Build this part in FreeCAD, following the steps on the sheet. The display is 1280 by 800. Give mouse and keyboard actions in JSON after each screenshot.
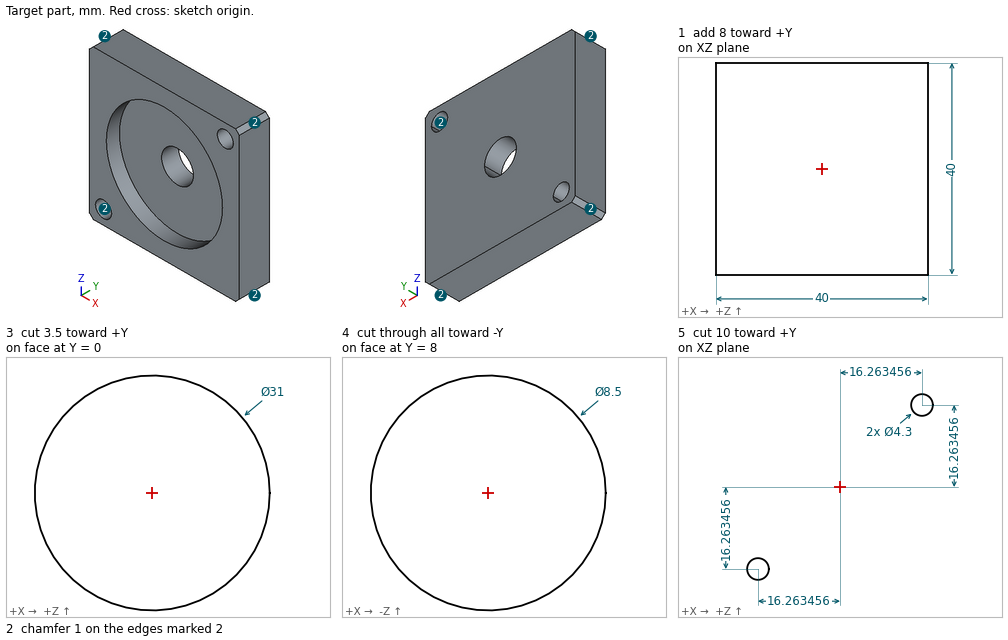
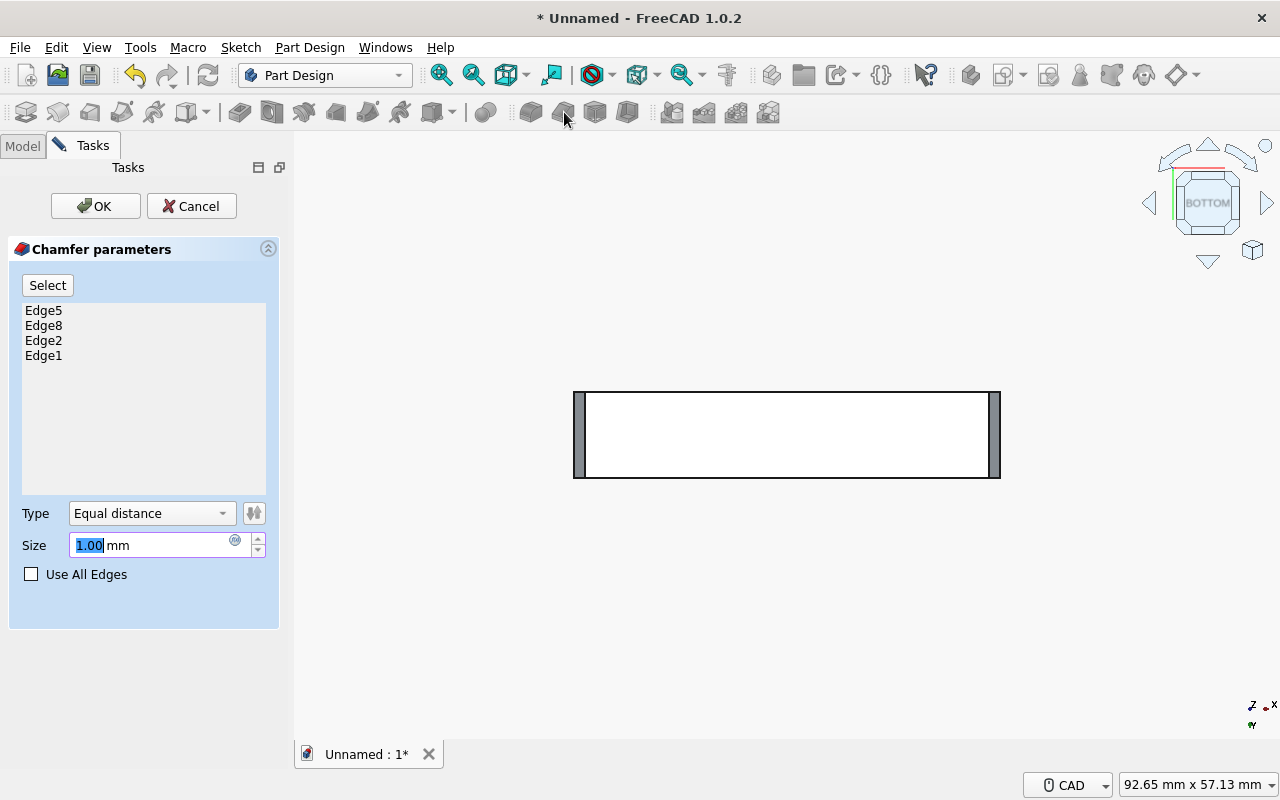
{"action": "type", "text": "1"}
{"action": "key", "text": "Tab"}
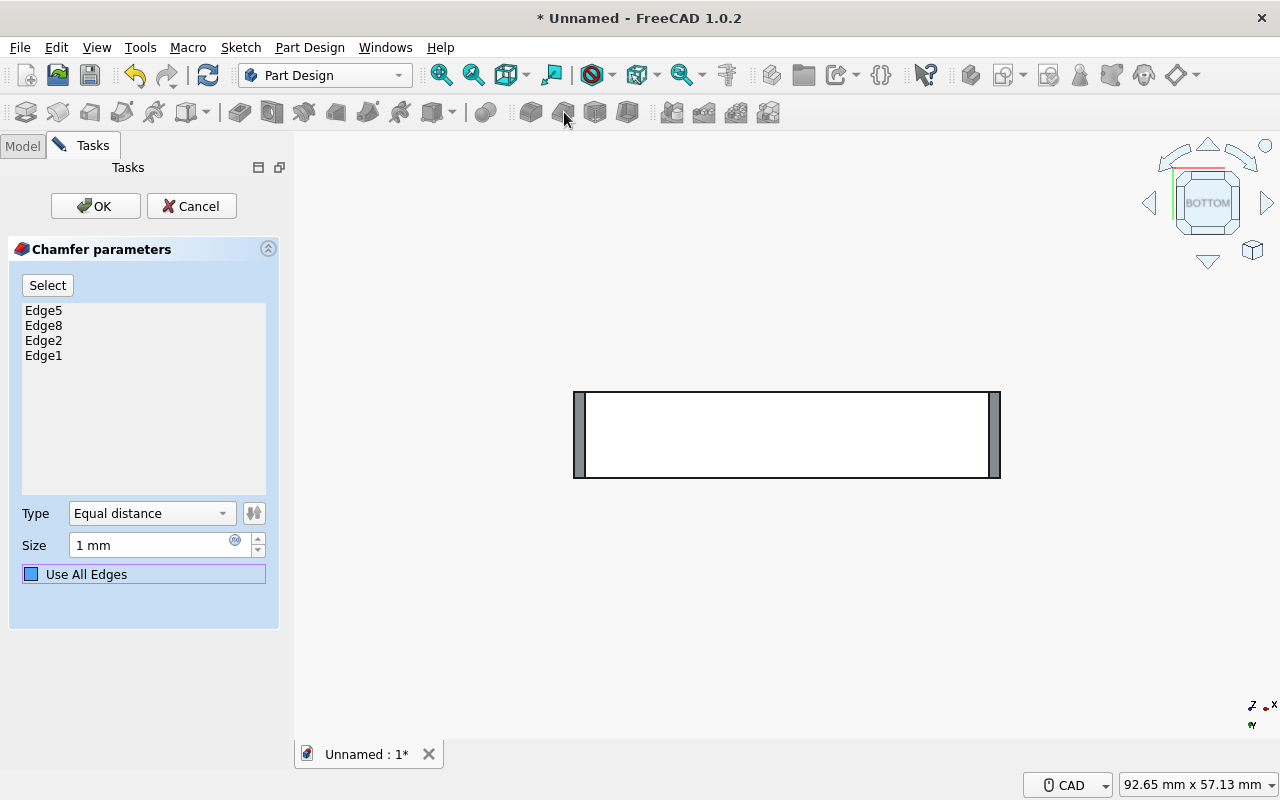
{"action": "left_click", "coordinate": [96, 206]}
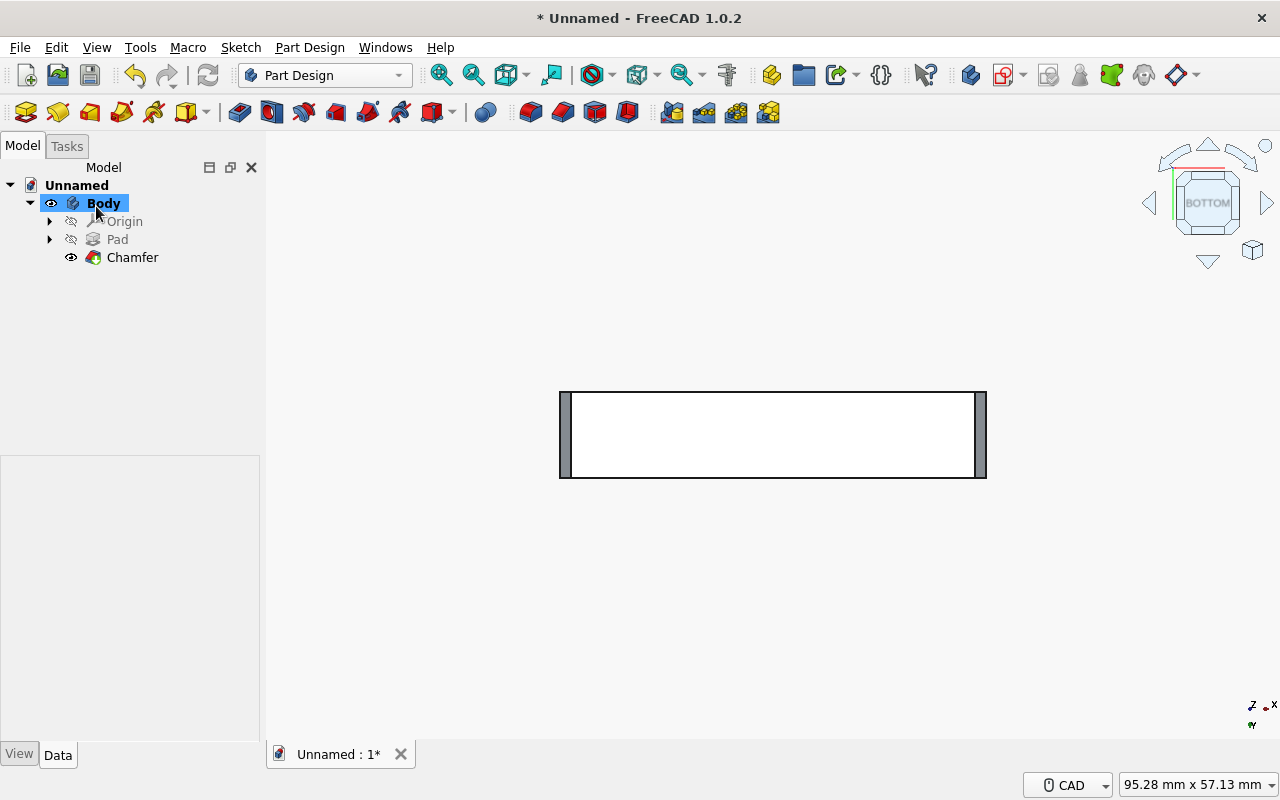
{"action": "left_click", "coordinate": [442, 76]}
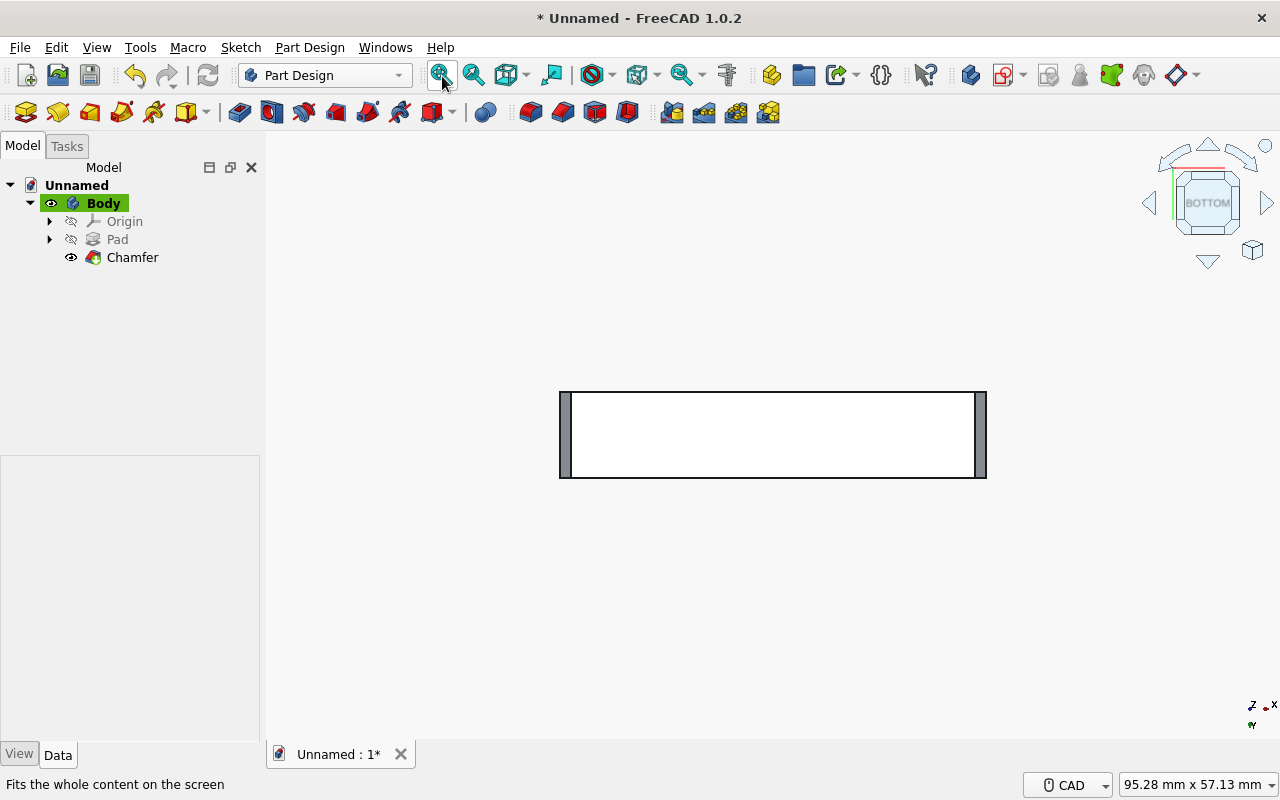
{"action": "key", "text": "0"}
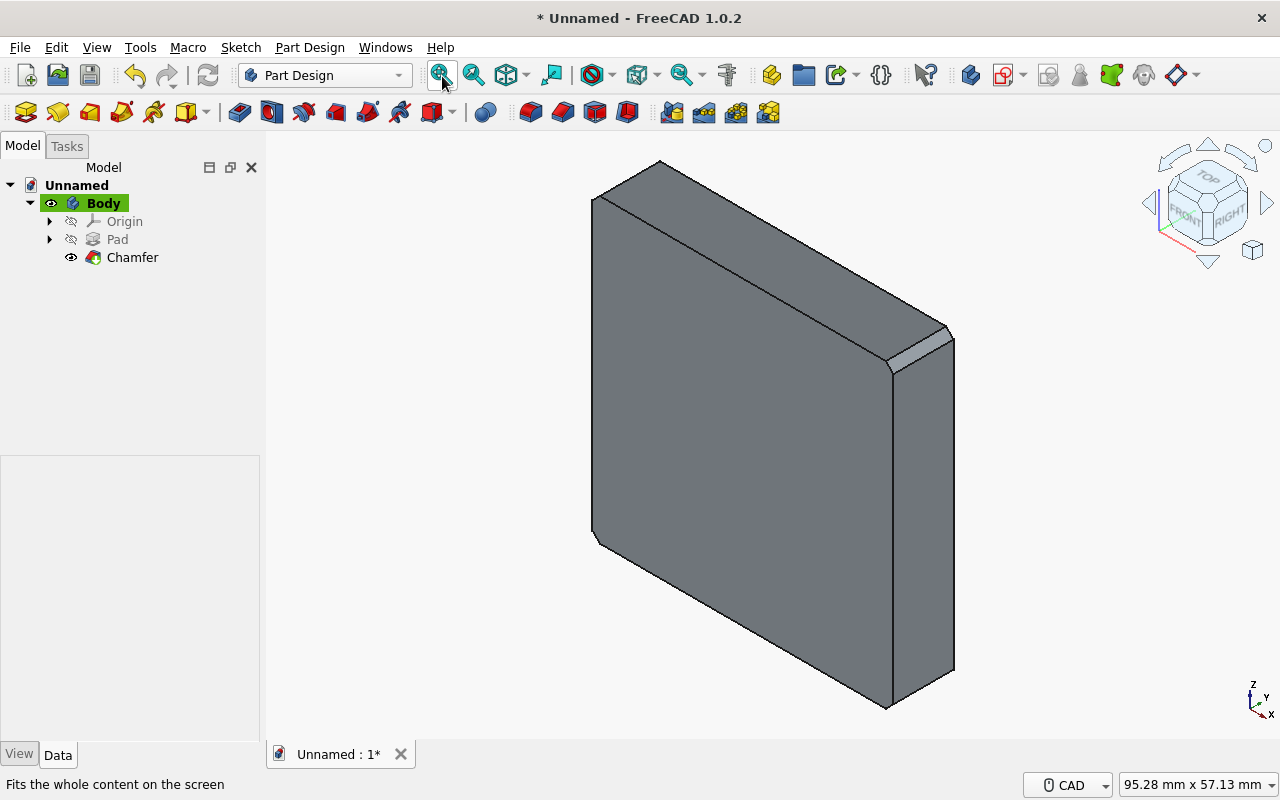
{"action": "left_click", "coordinate": [743, 451]}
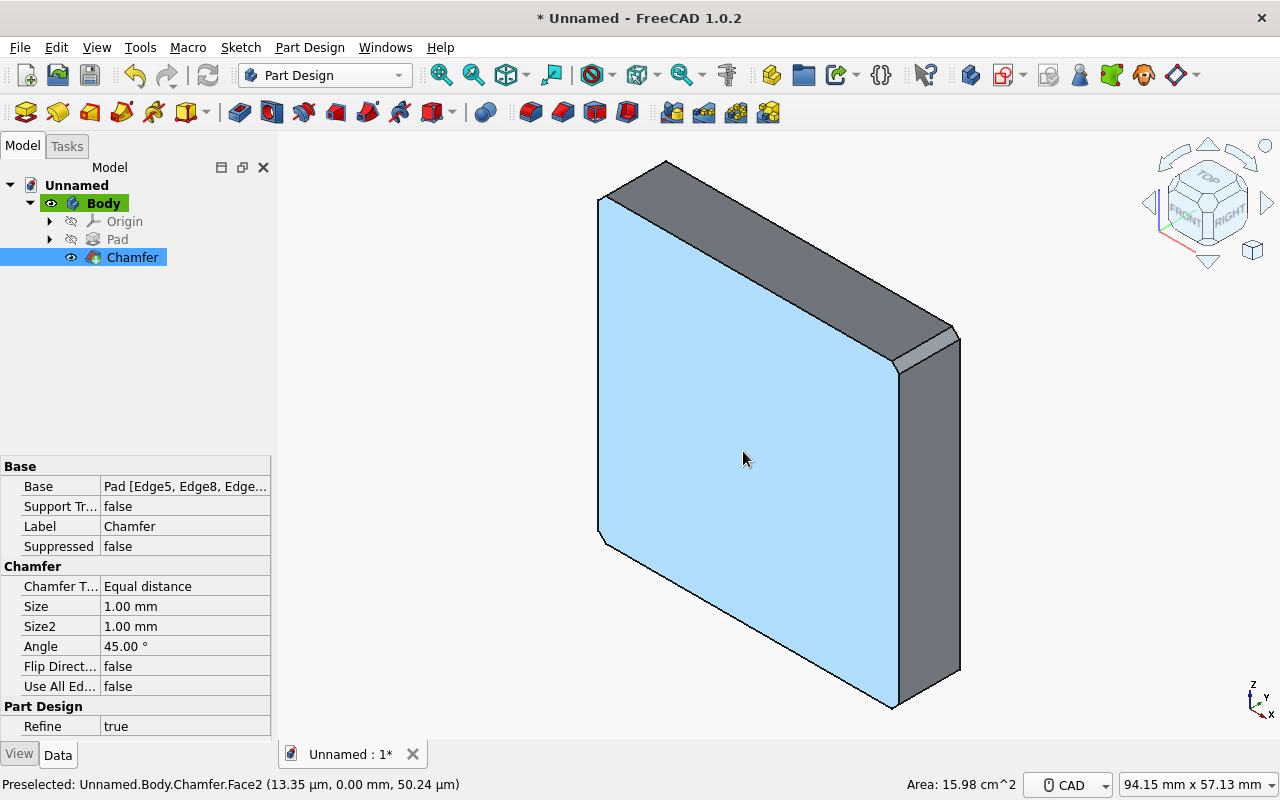
{"action": "left_click", "coordinate": [1004, 76]}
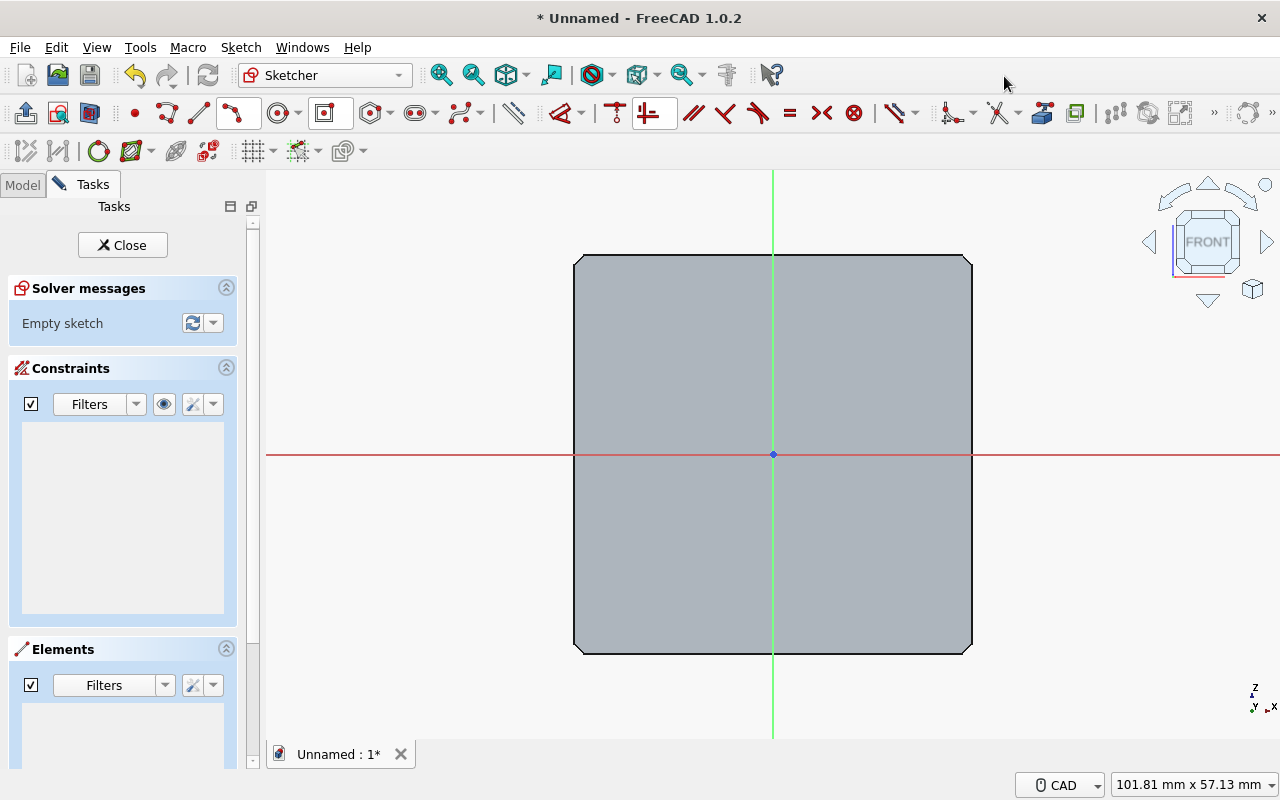
{"action": "left_click", "coordinate": [278, 114]}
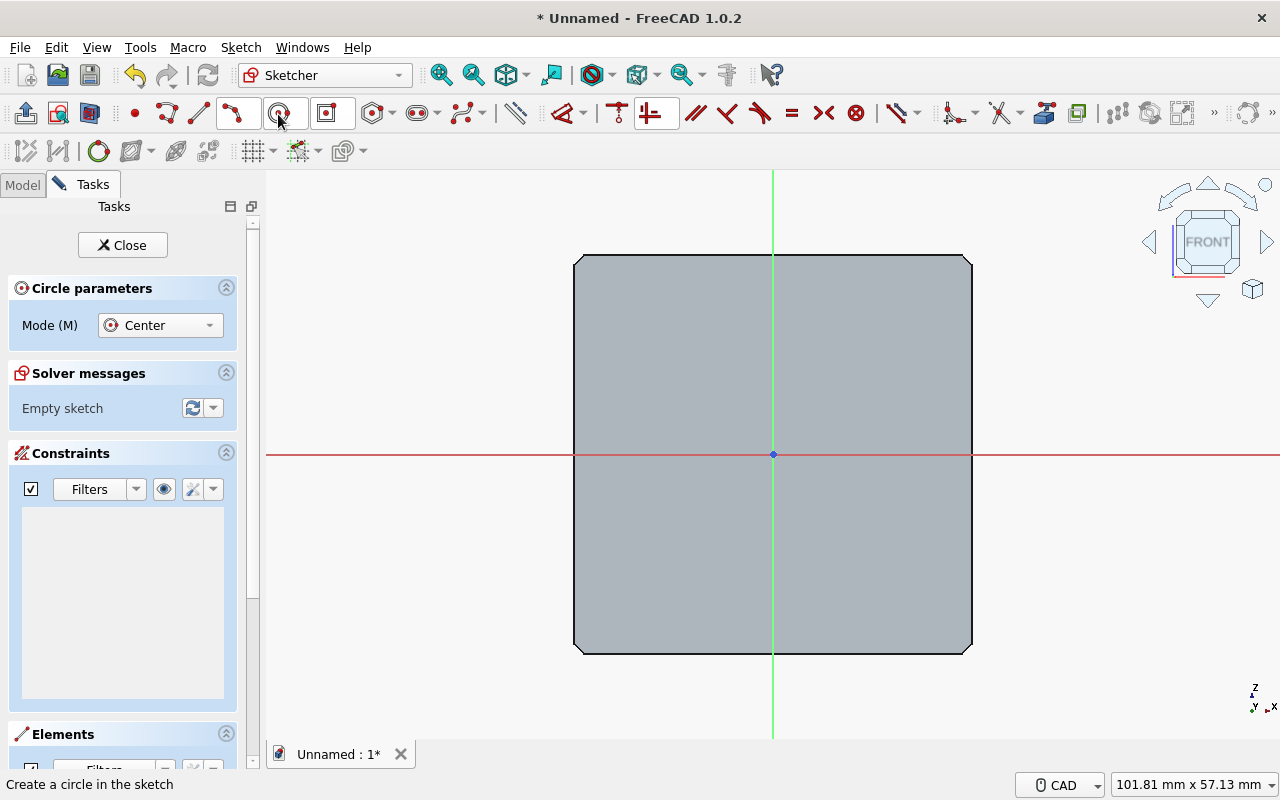
{"action": "left_click", "coordinate": [773, 455]}
{"action": "left_click", "coordinate": [882, 345]}
{"action": "key", "text": "Escape"}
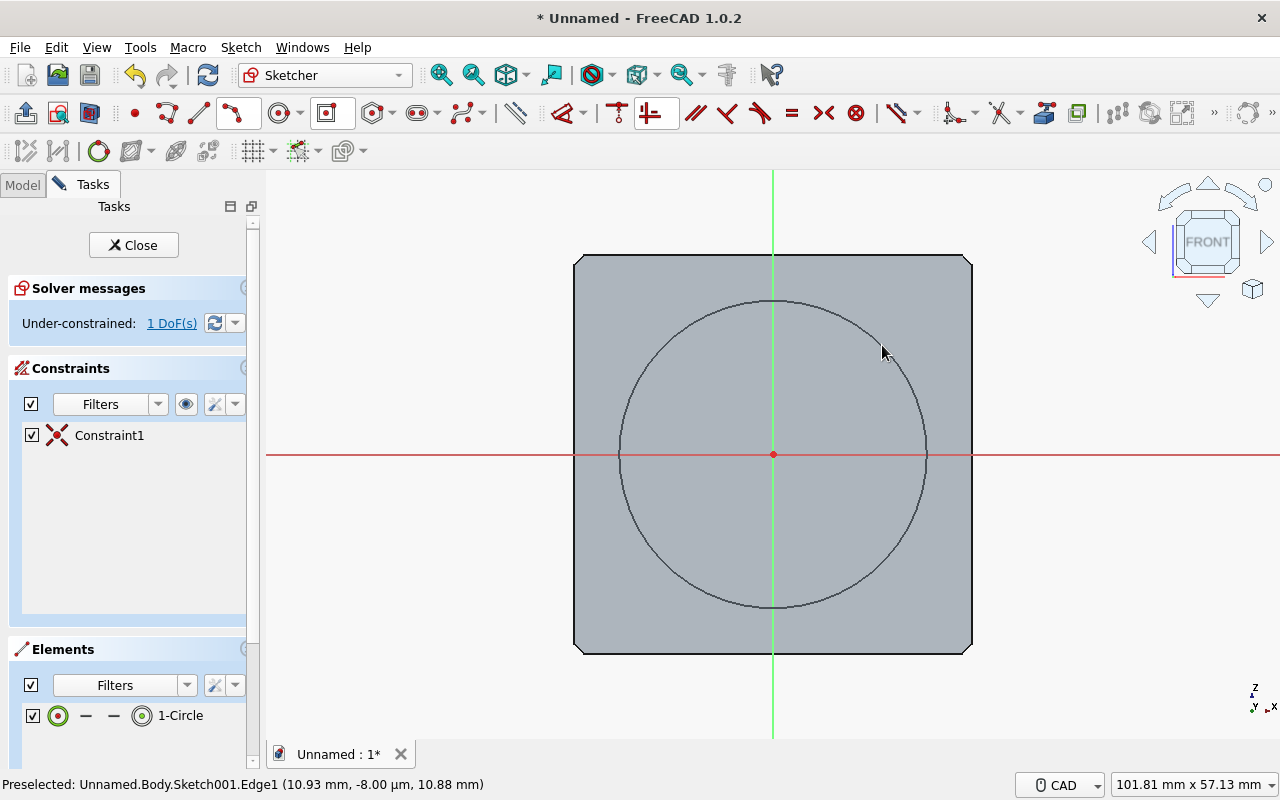
{"action": "left_click", "coordinate": [562, 114]}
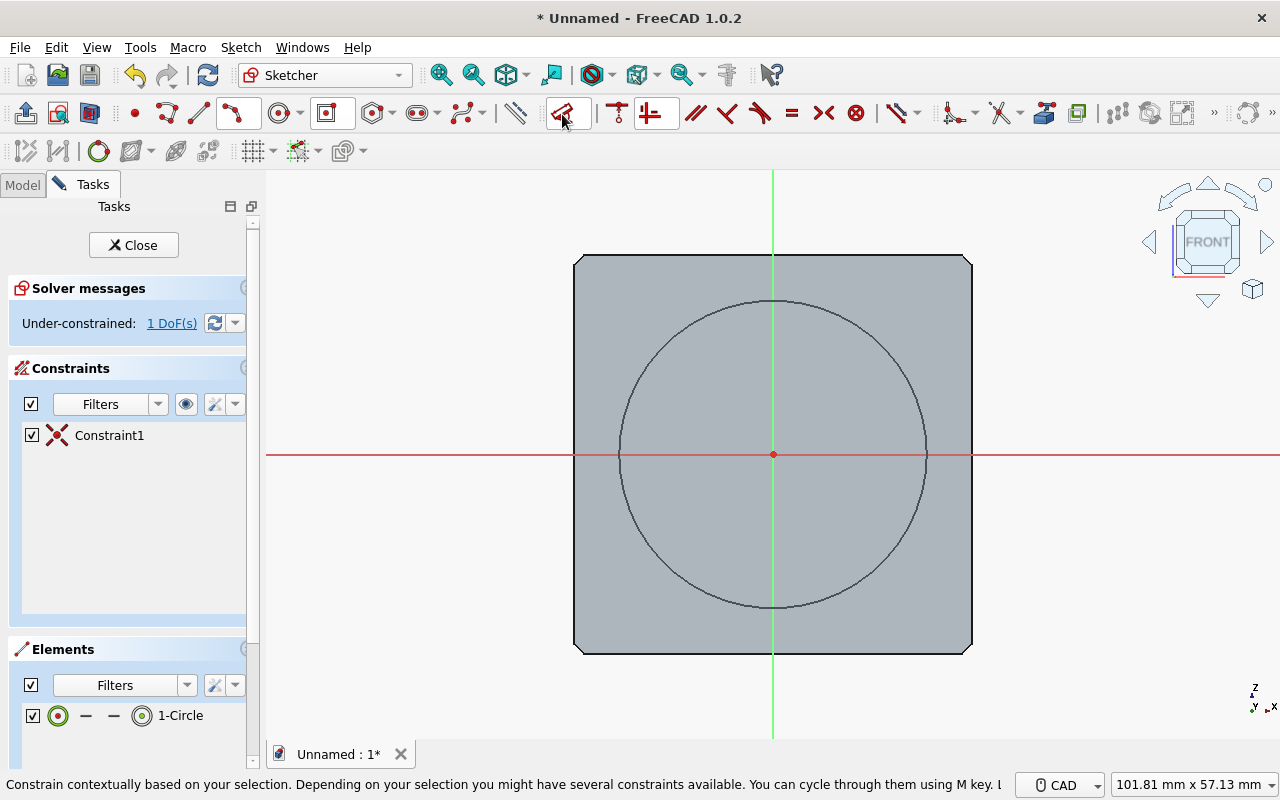
{"action": "left_click", "coordinate": [881, 345]}
{"action": "left_click", "coordinate": [903, 322]}